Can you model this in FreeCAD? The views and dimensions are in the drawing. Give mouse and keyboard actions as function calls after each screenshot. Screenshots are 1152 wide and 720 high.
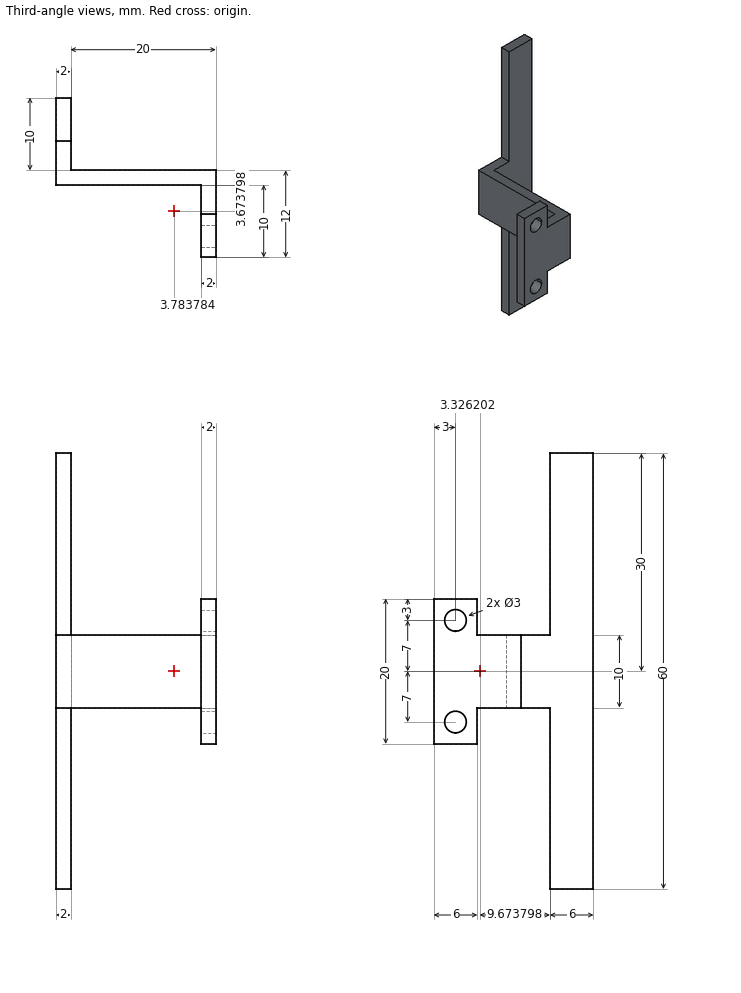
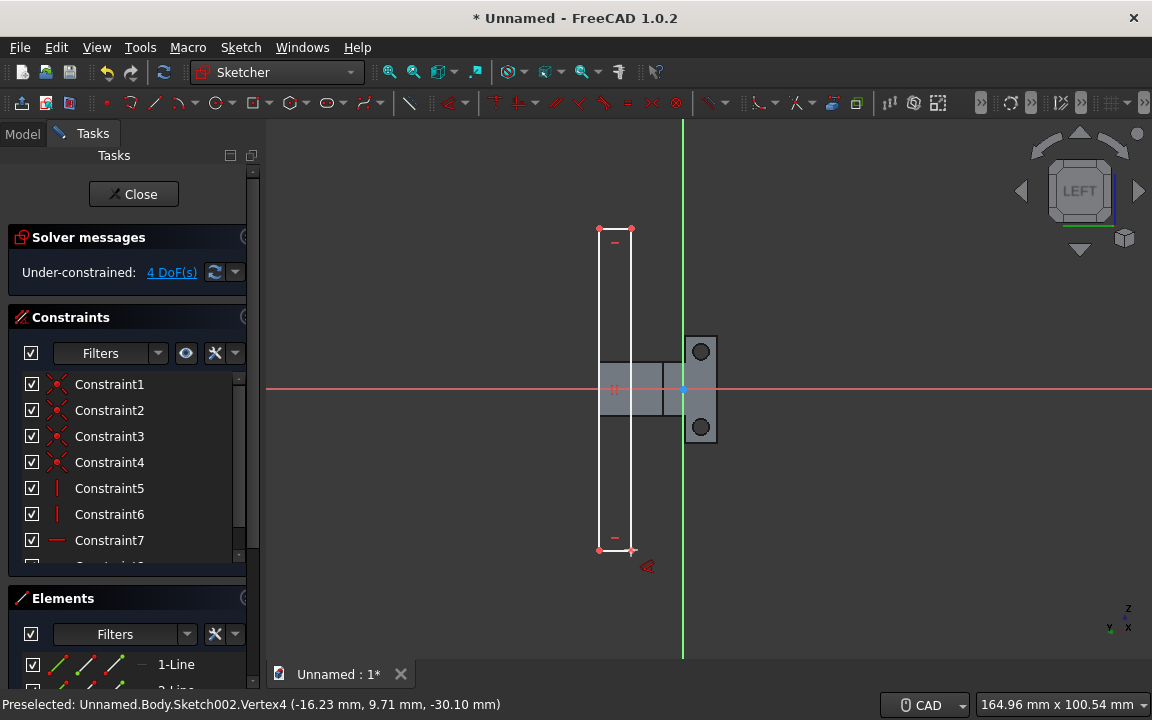
scroll(609, 551, up, 2)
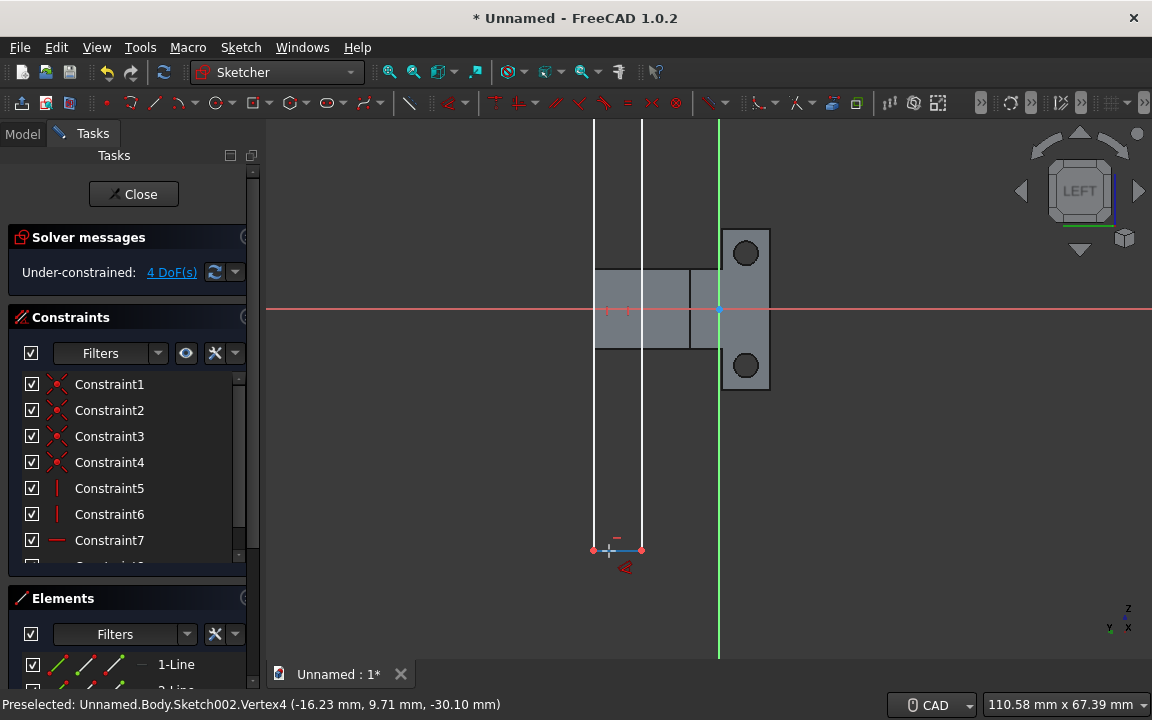
click(608, 551)
click(618, 585)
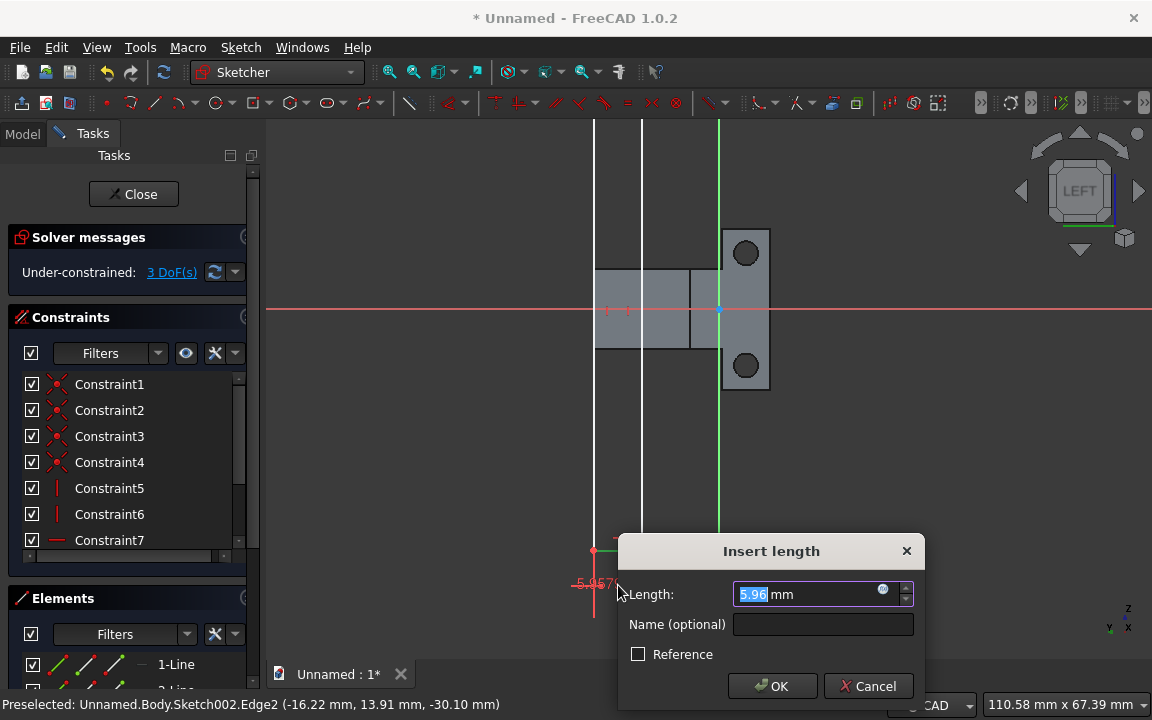
text(6)
key(Return)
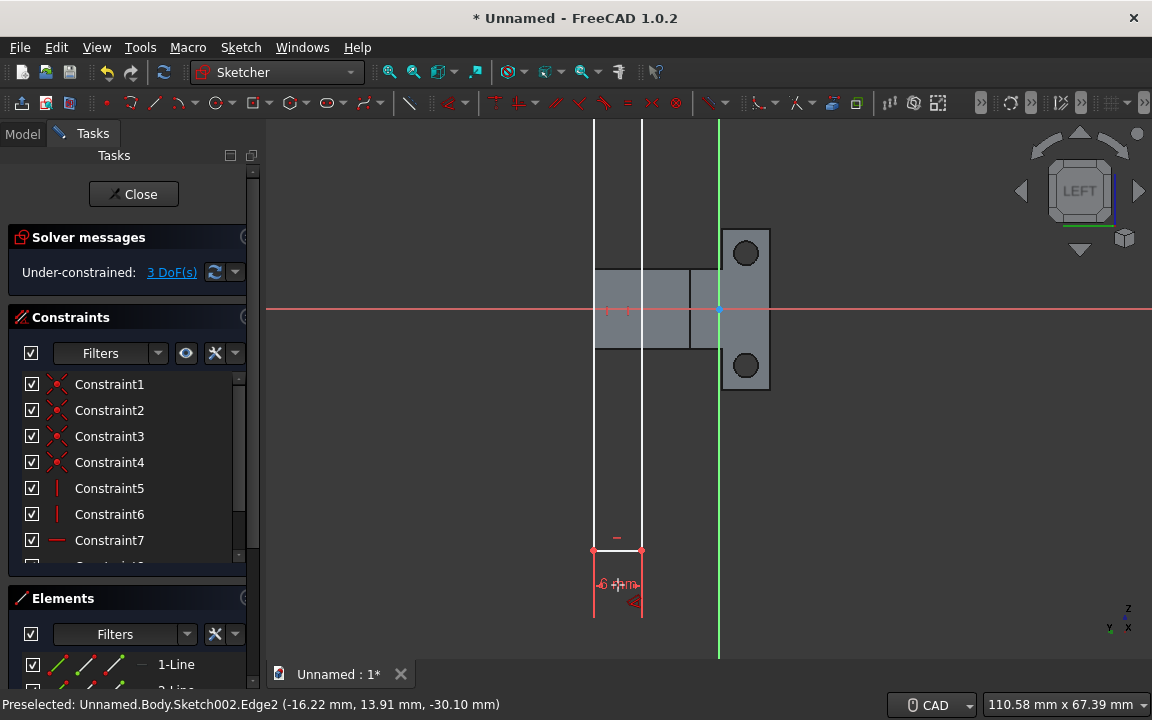
click(594, 214)
click(560, 349)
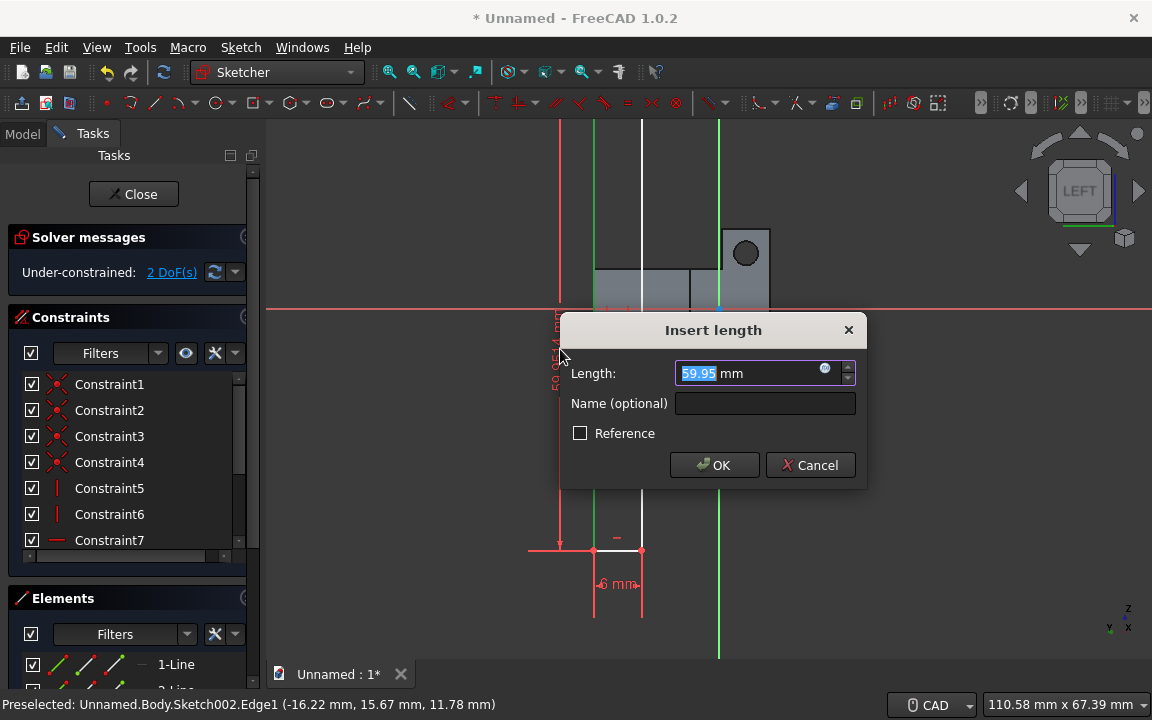
text(60)
key(Return)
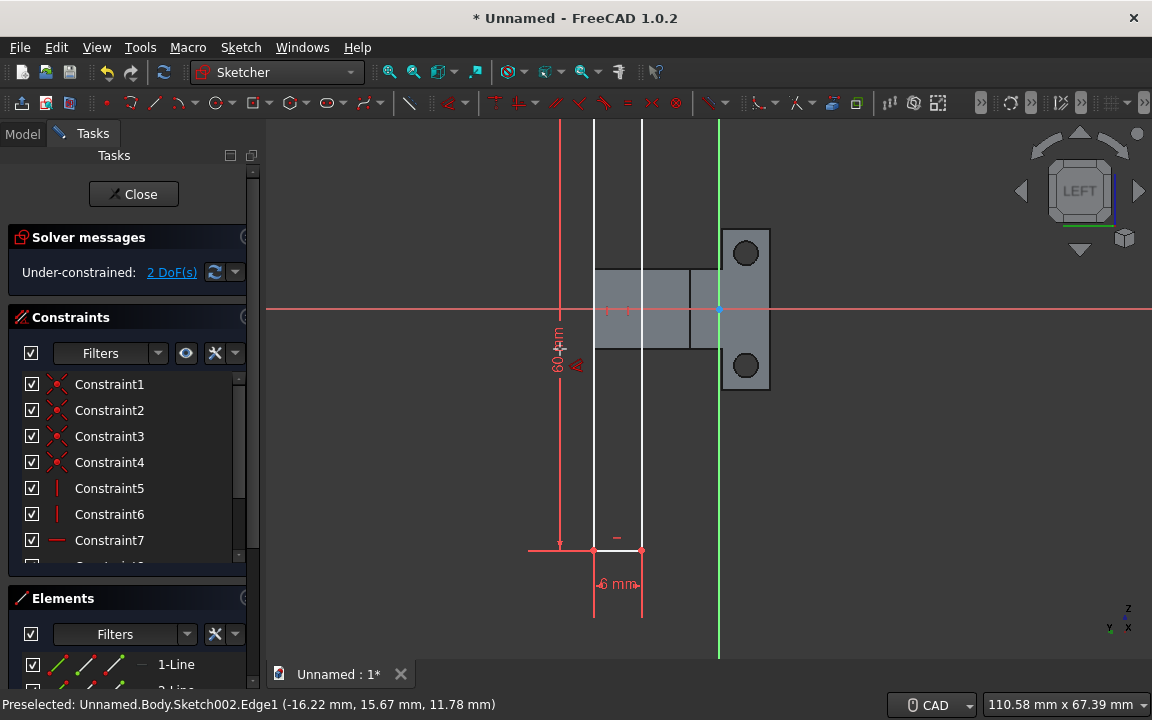
scroll(608, 551, down, 2)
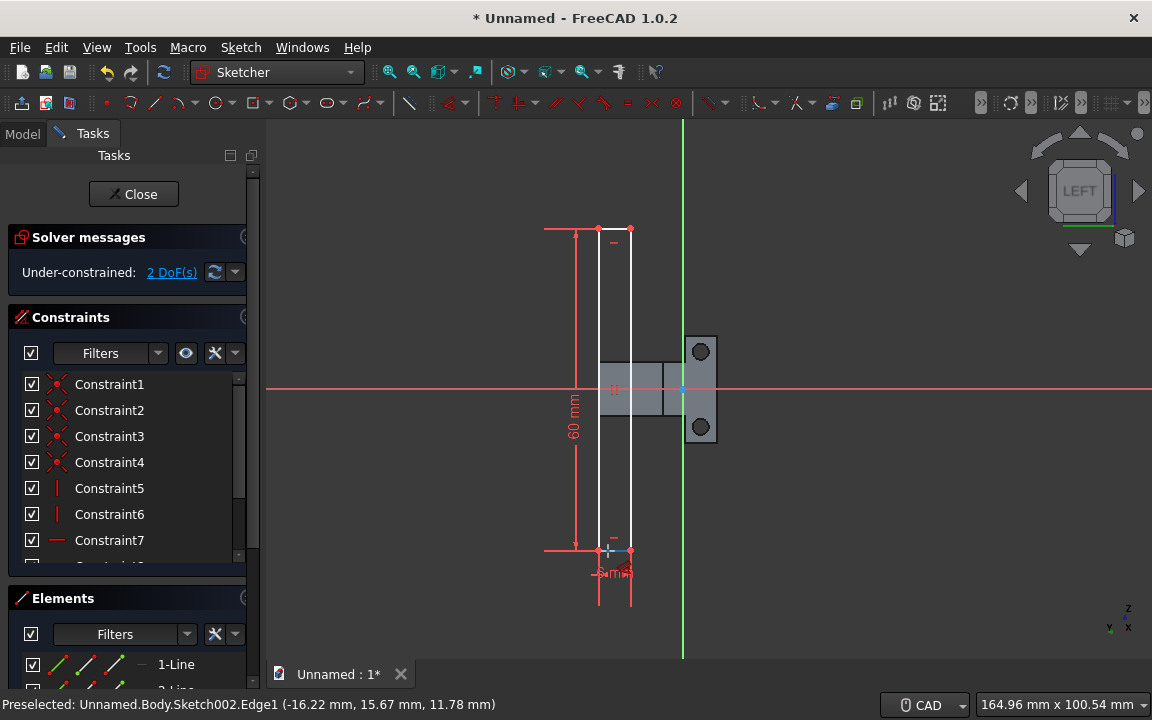
click(599, 229)
click(717, 309)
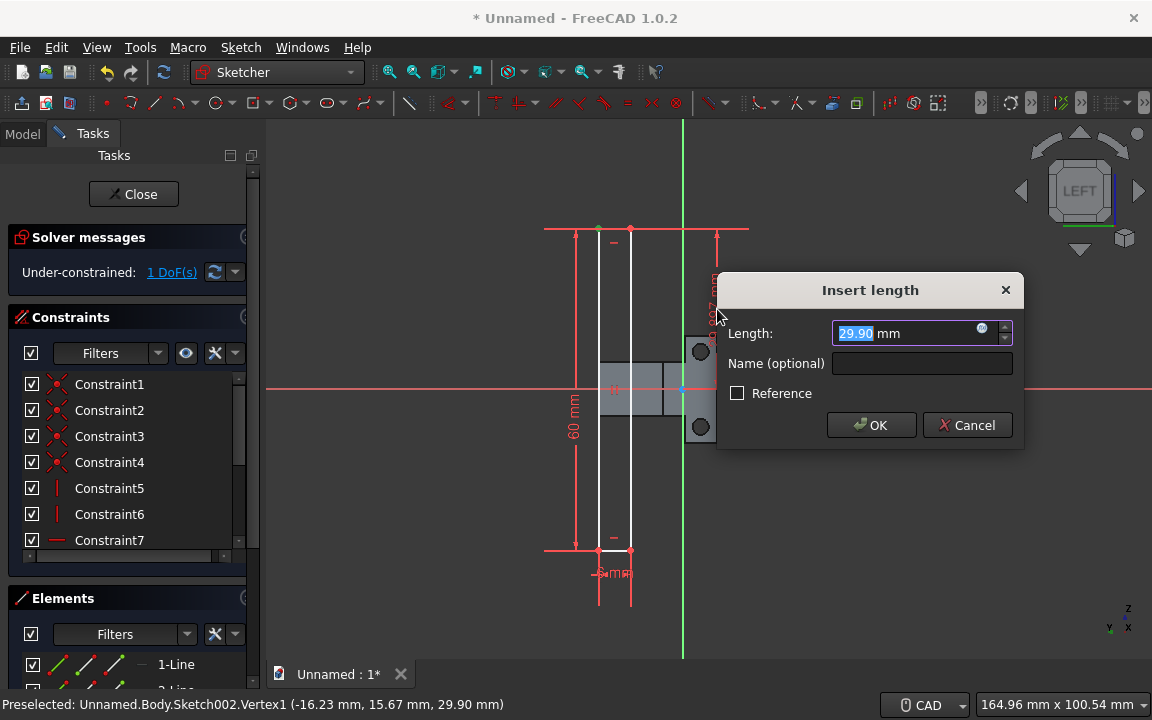
text(30)
key(Return)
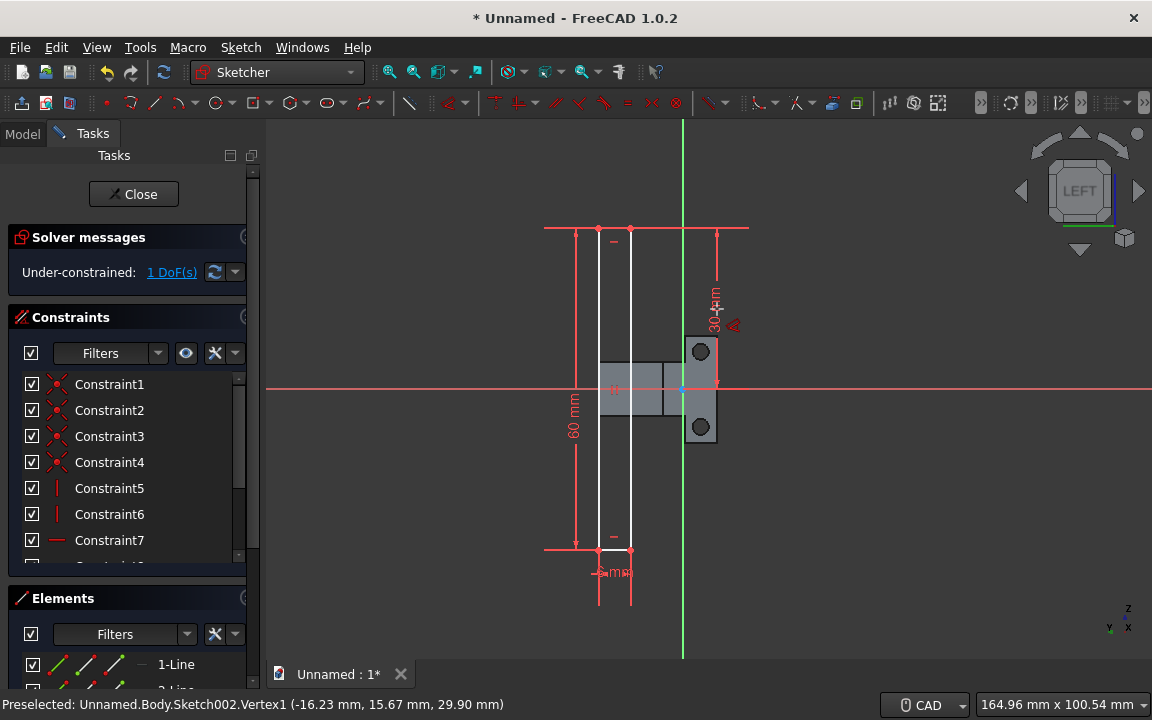
click(631, 550)
click(657, 355)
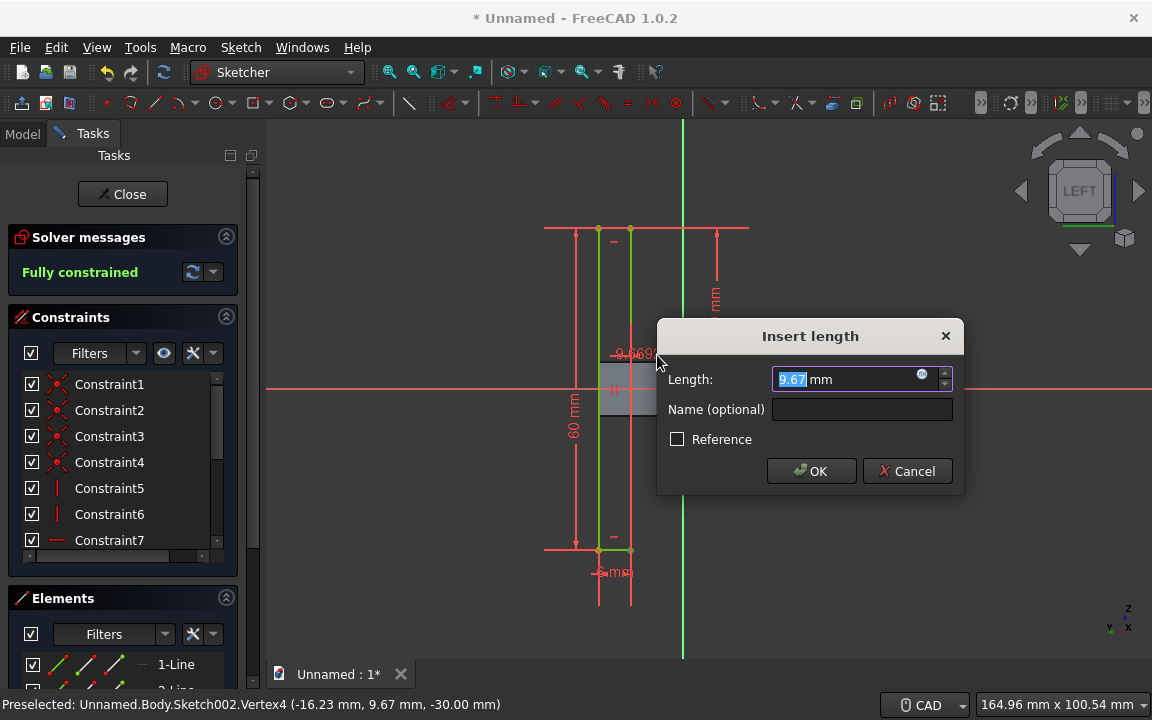
text(9.673798)
key(Return)
key(Escape)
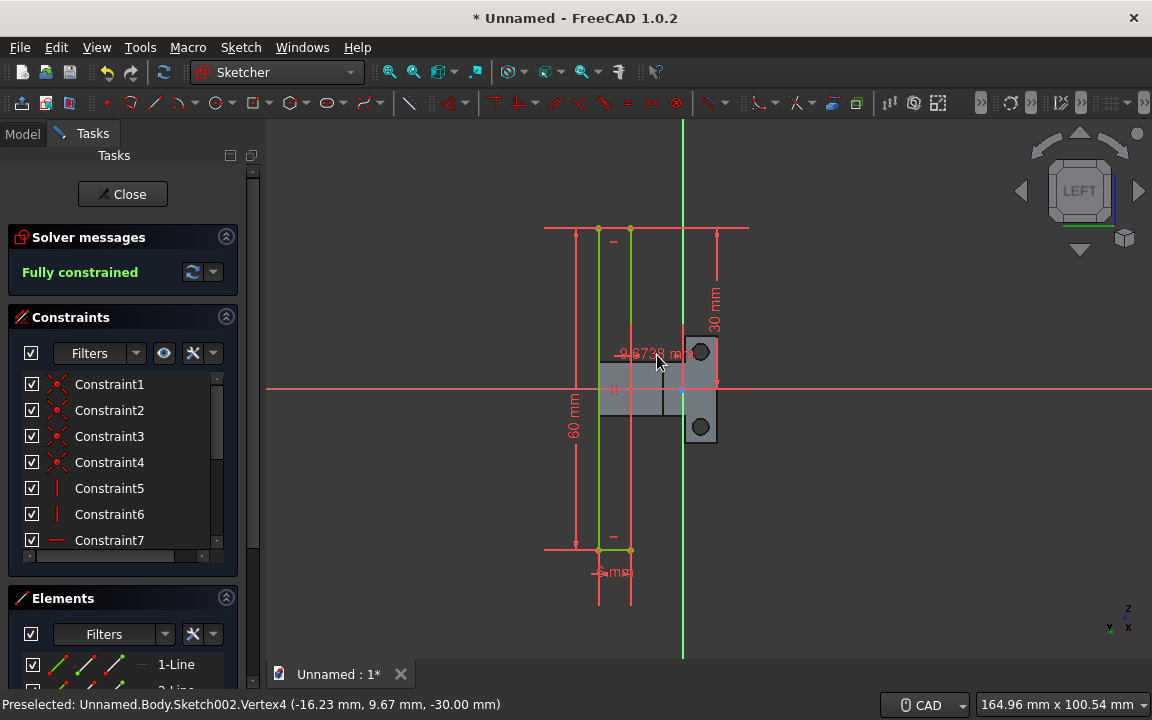
click(123, 194)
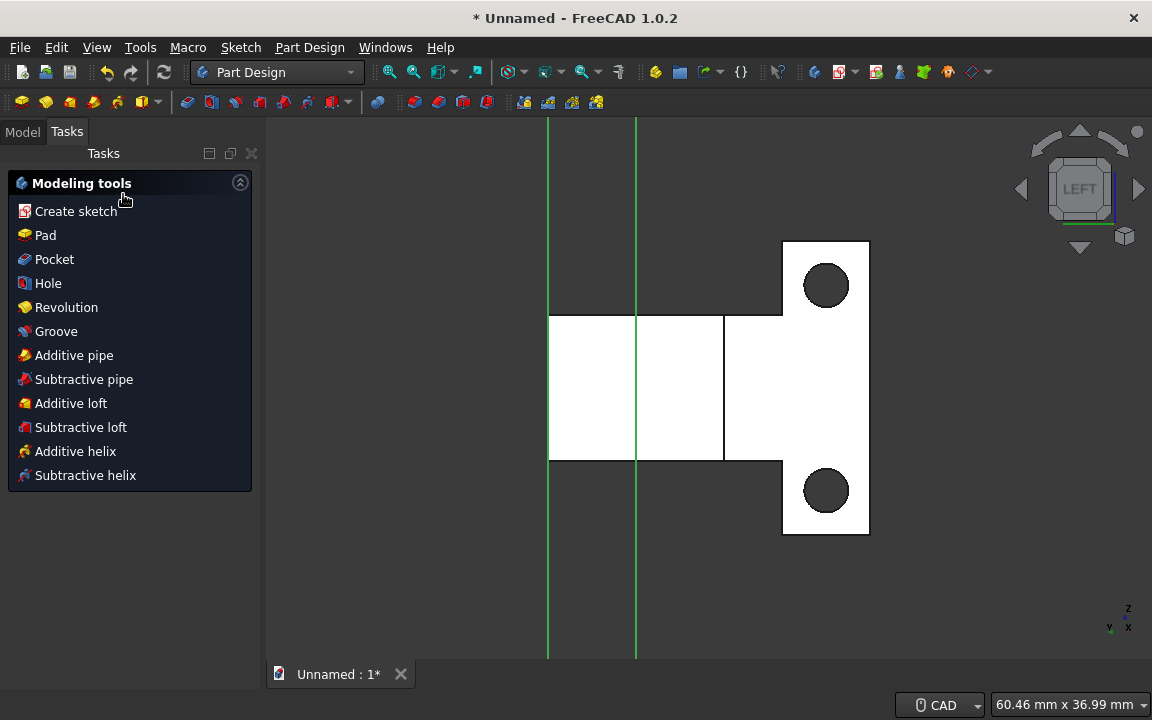
click(22, 102)